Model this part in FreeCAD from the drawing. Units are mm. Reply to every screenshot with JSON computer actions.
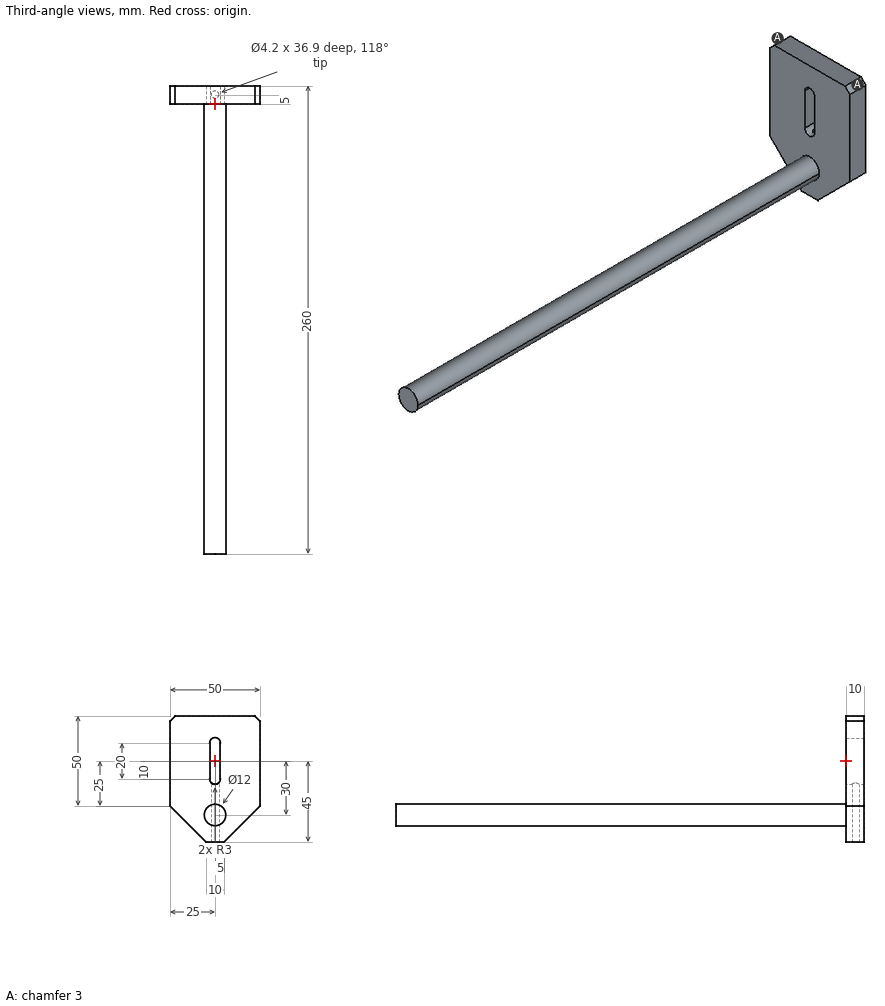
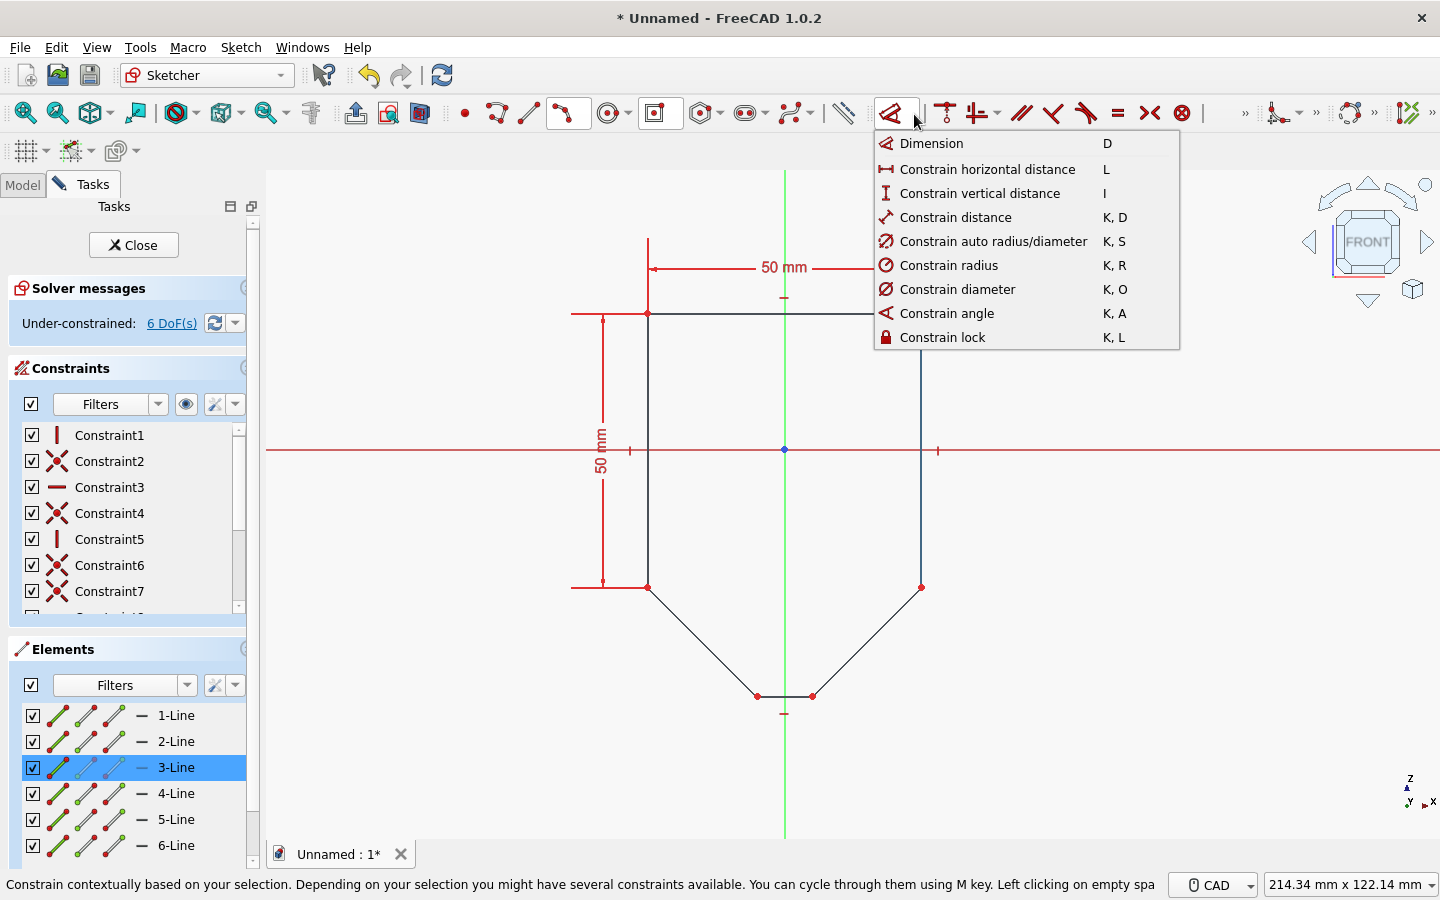
{"action": "left_click", "coordinate": [1027, 193]}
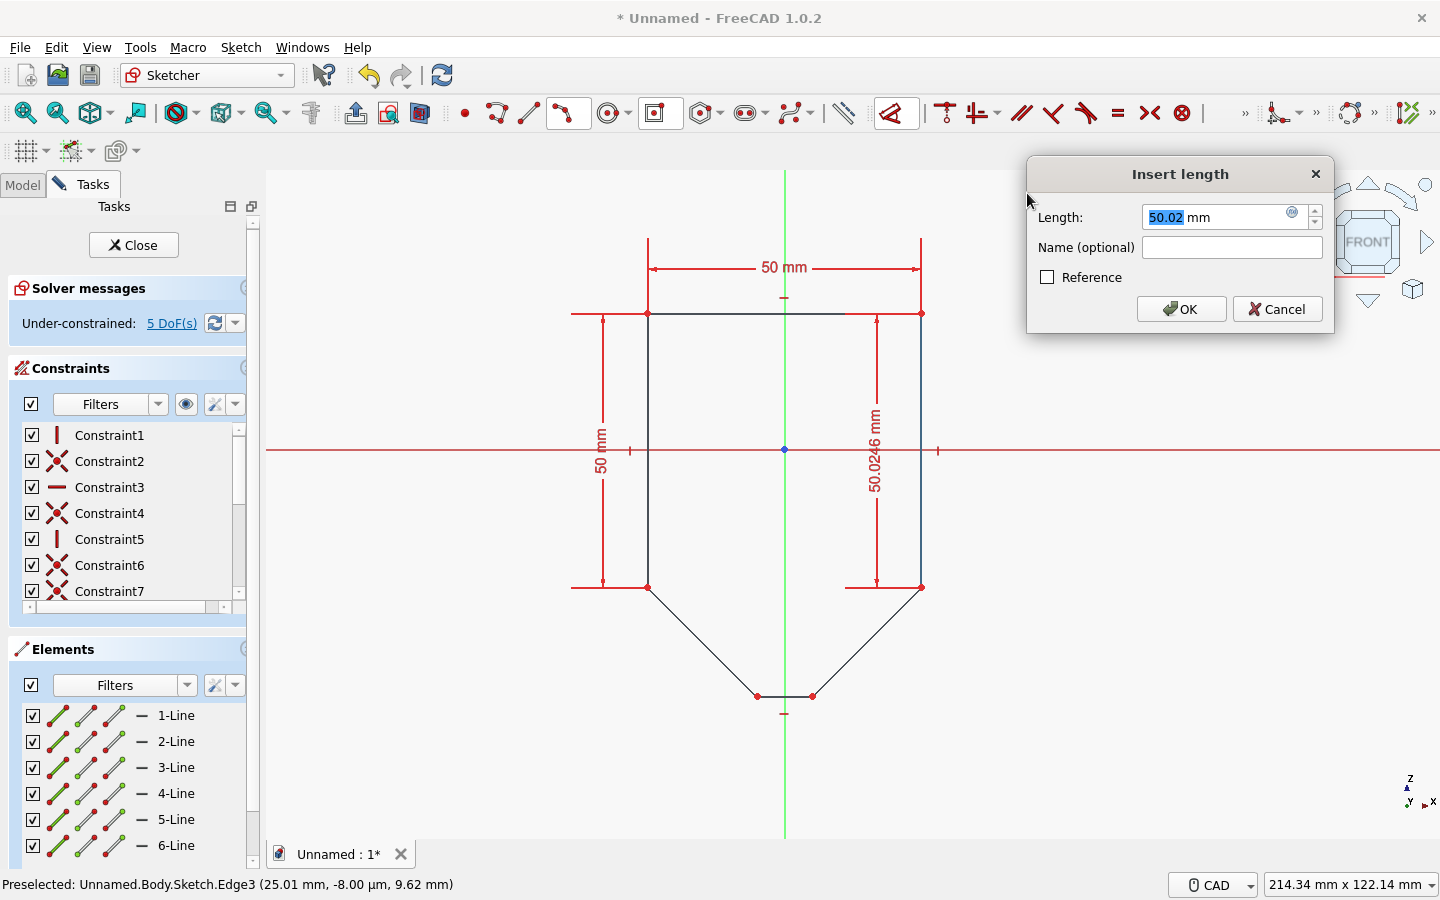
{"action": "type", "text": "50"}
{"action": "key", "text": "Return"}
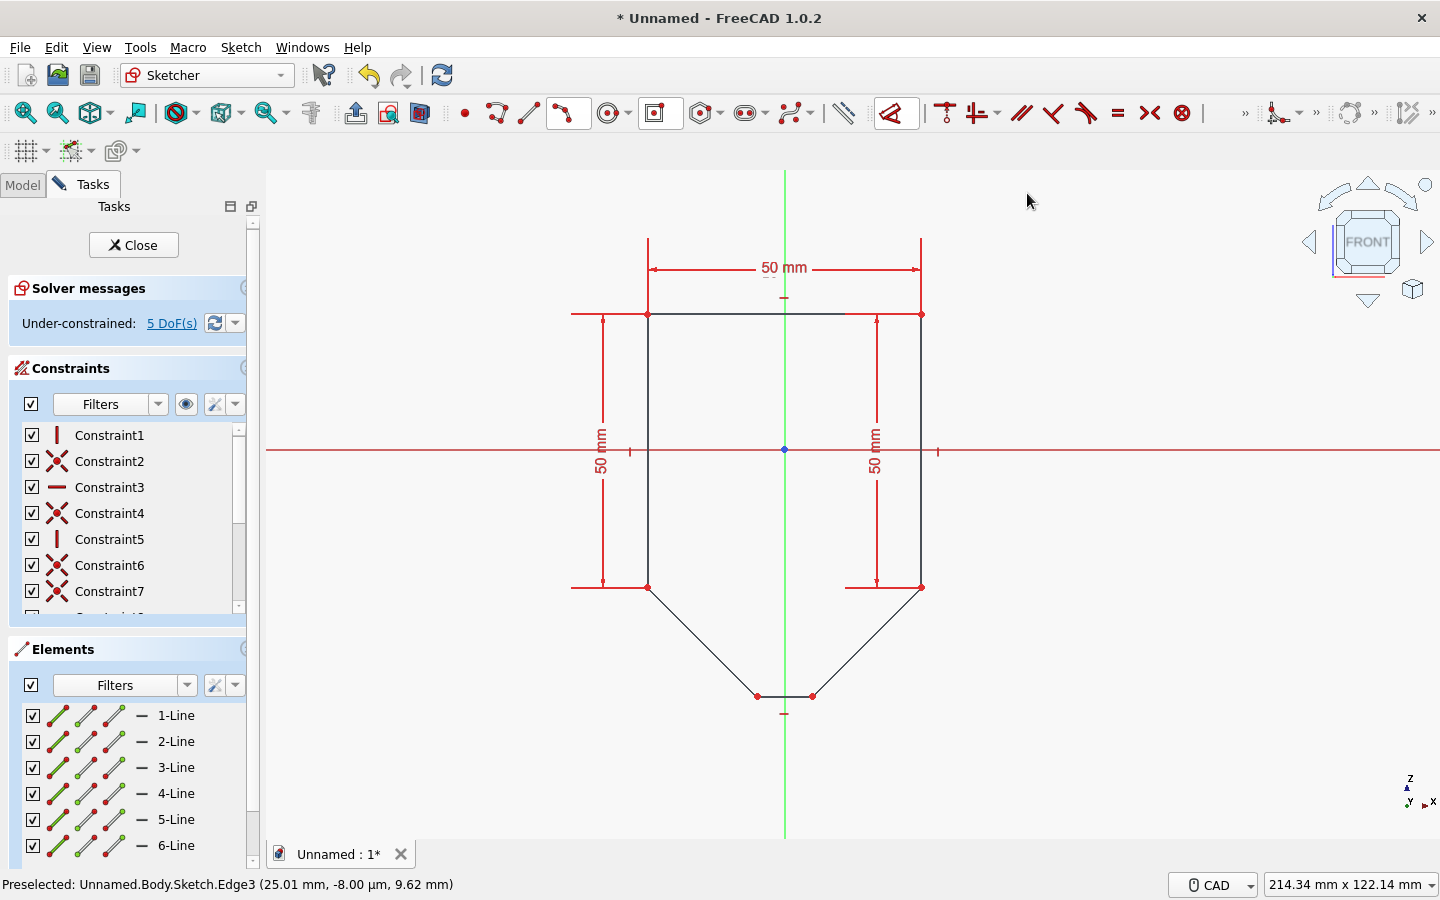
{"action": "scroll", "coordinate": [796, 697], "scroll_direction": "up", "scroll_amount": 2}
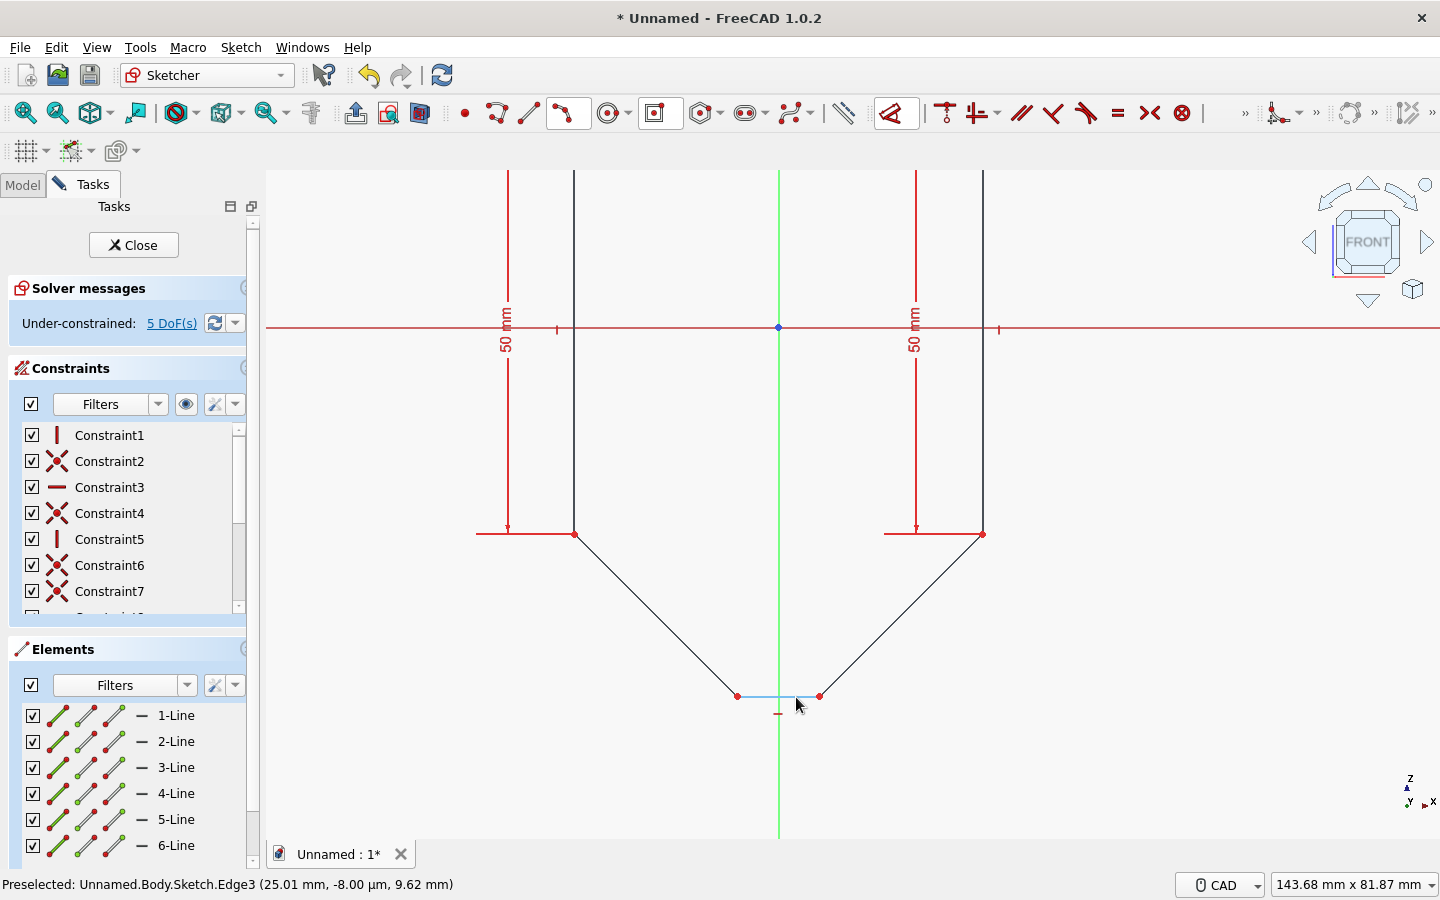
{"action": "left_click", "coordinate": [795, 697]}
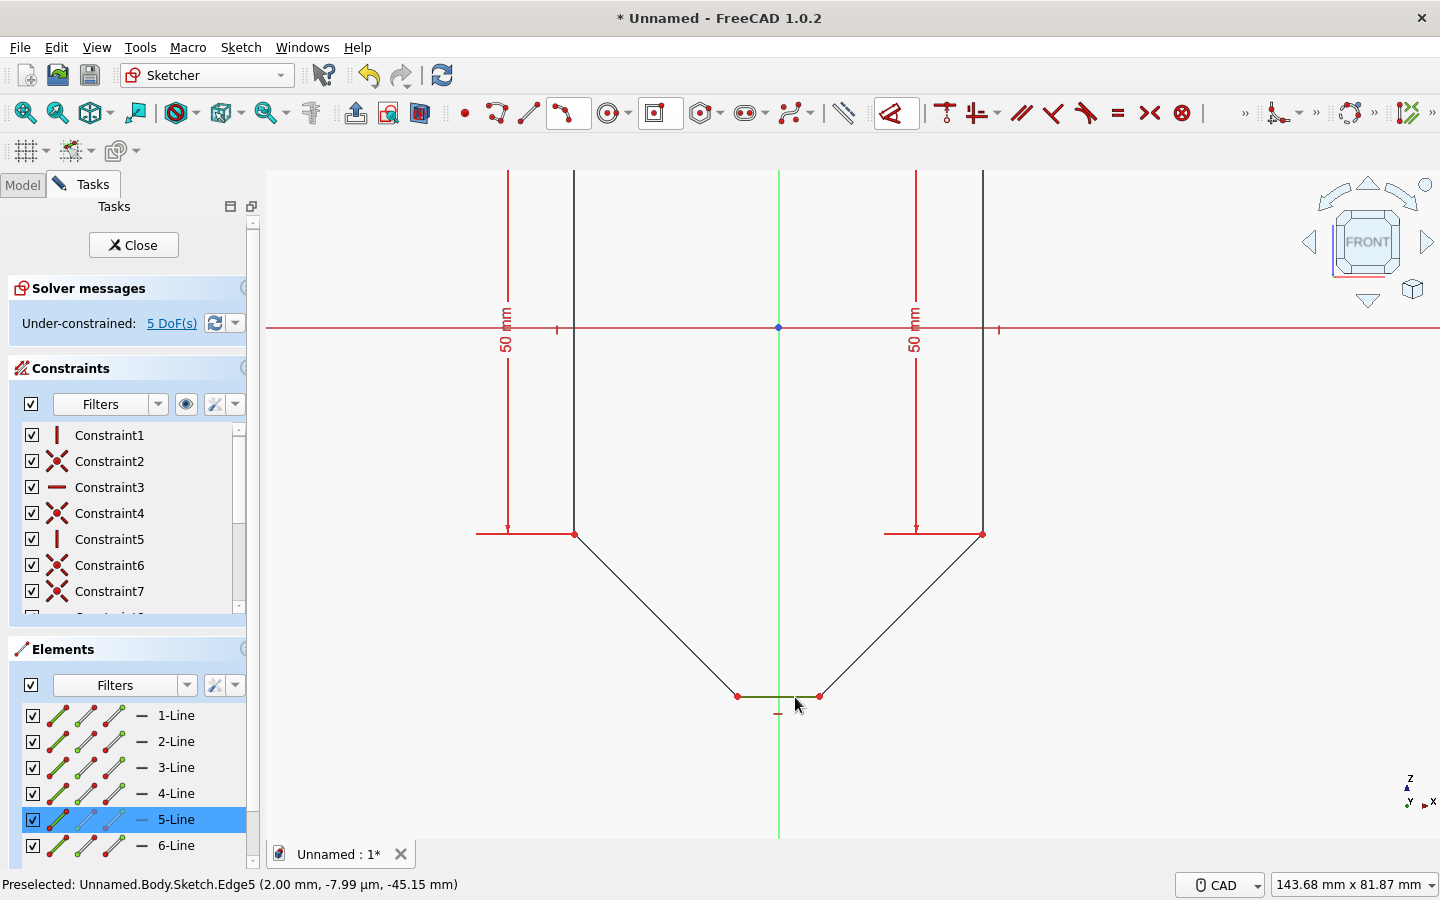
{"action": "left_click", "coordinate": [914, 114]}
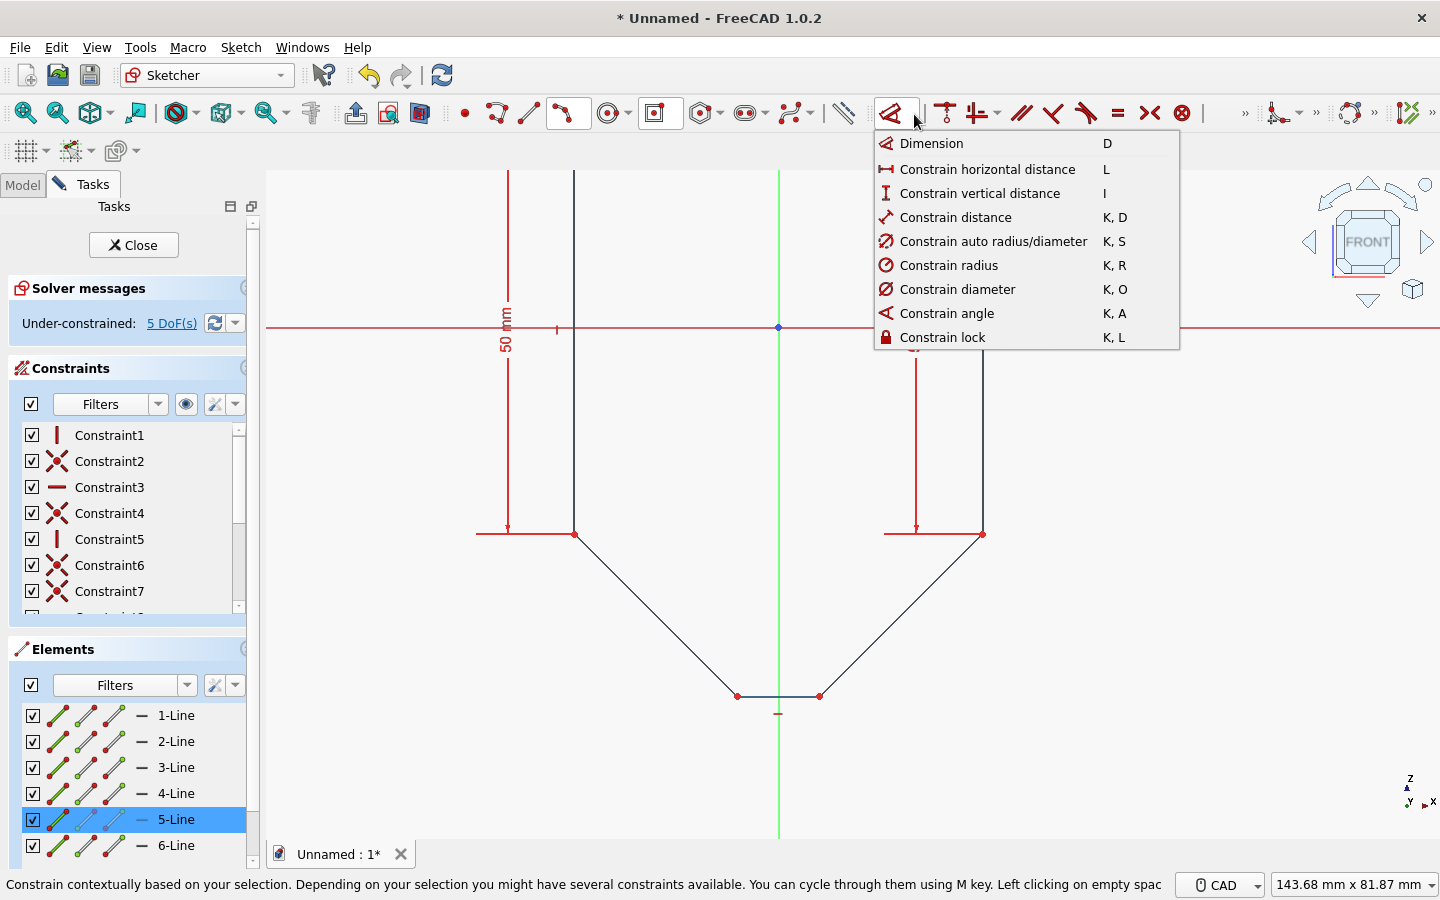
{"action": "left_click", "coordinate": [1027, 169]}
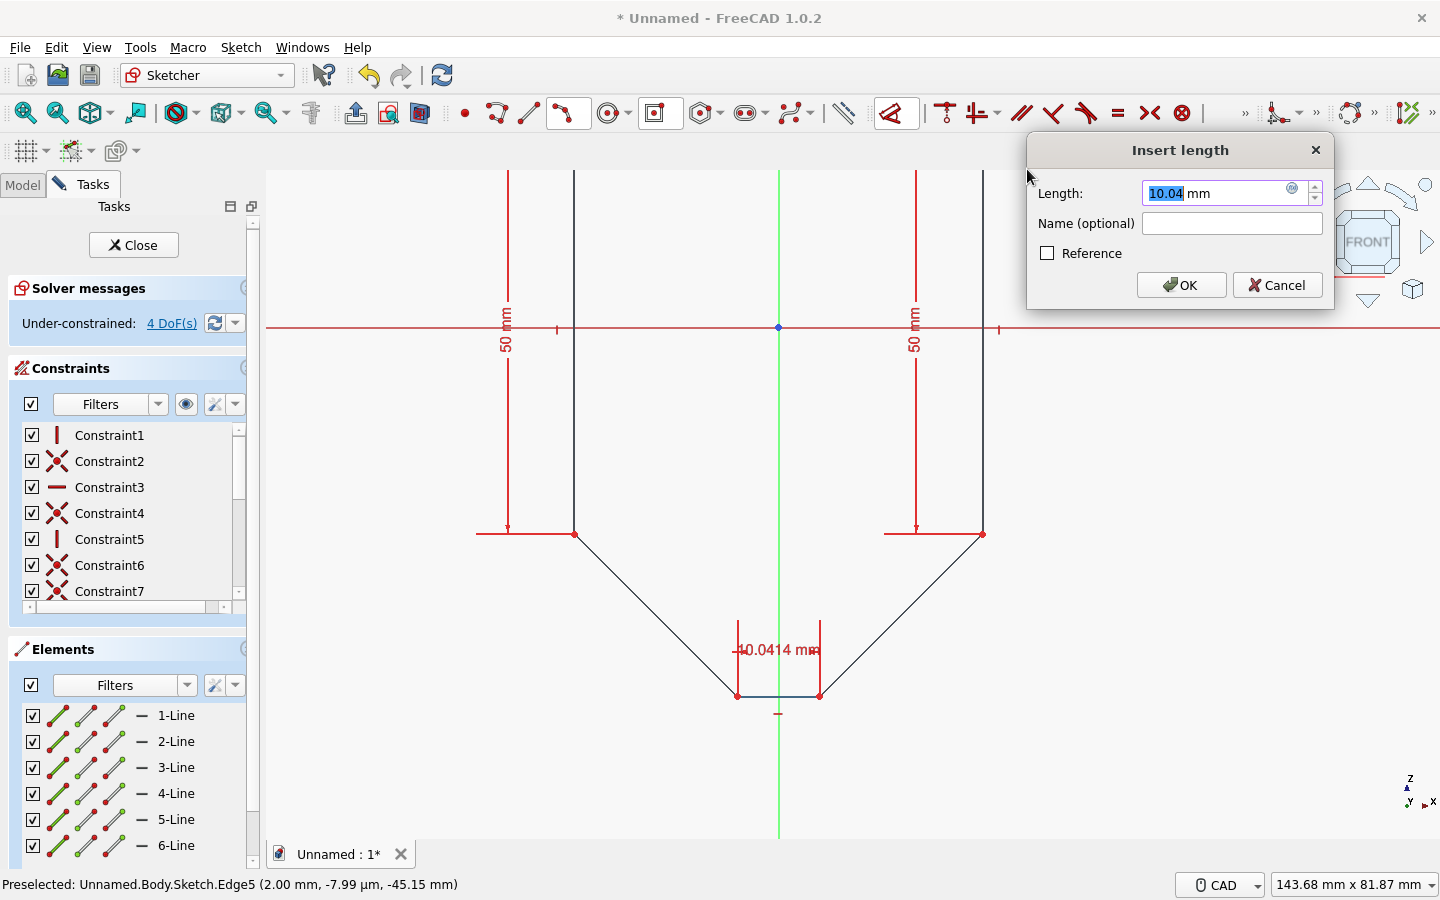
{"action": "type", "text": "10"}
{"action": "key", "text": "Return"}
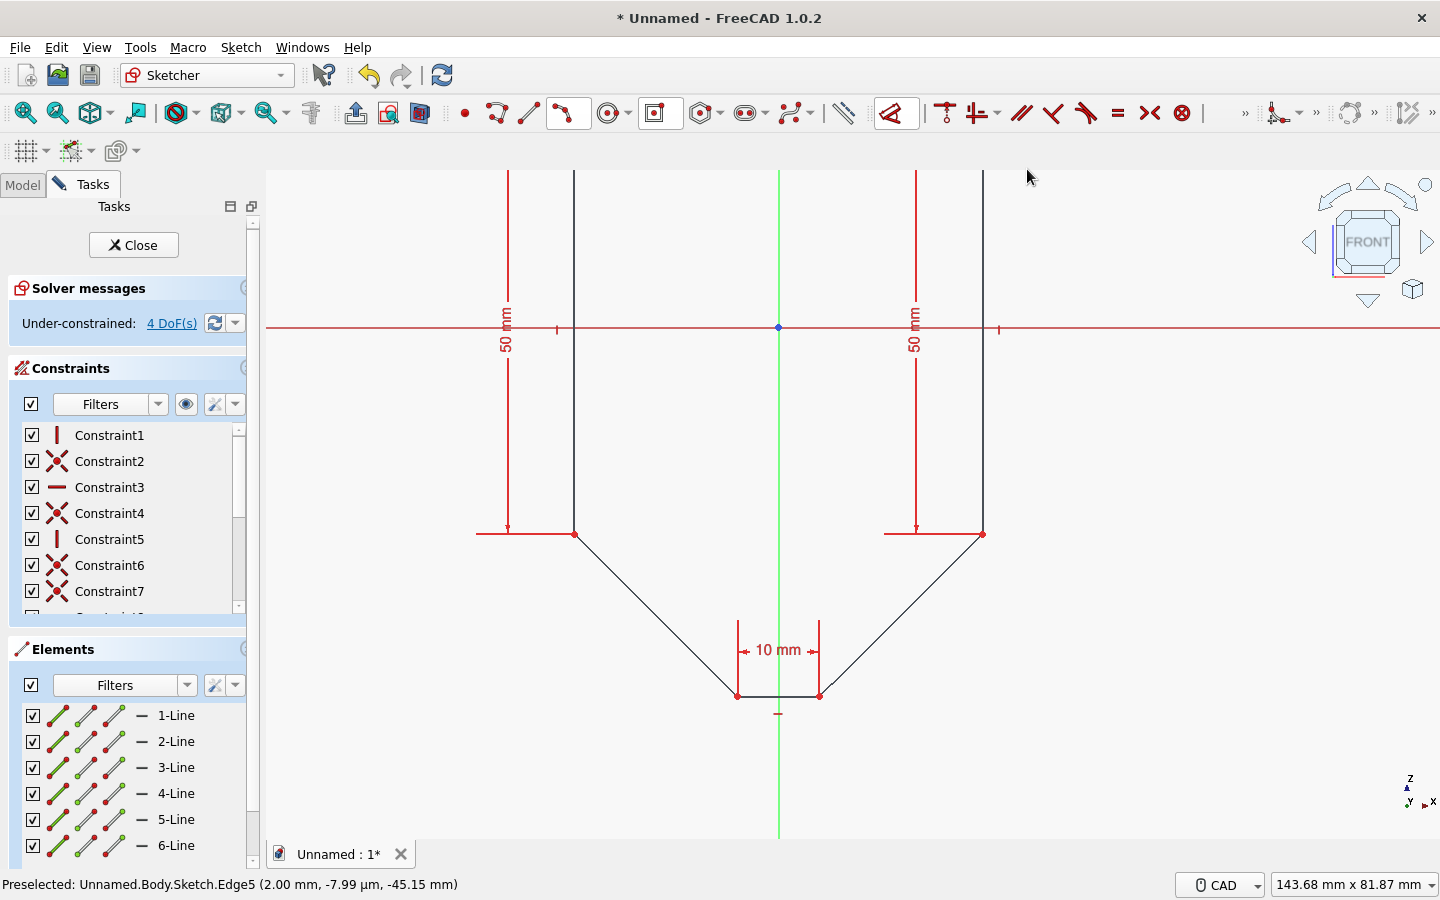
{"action": "left_click", "coordinate": [819, 697]}